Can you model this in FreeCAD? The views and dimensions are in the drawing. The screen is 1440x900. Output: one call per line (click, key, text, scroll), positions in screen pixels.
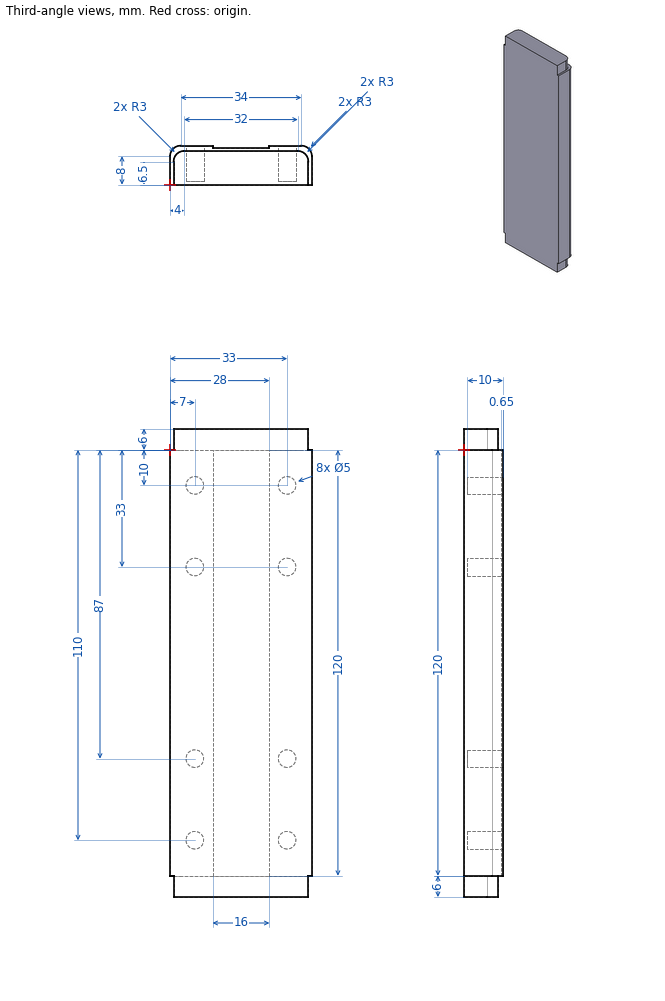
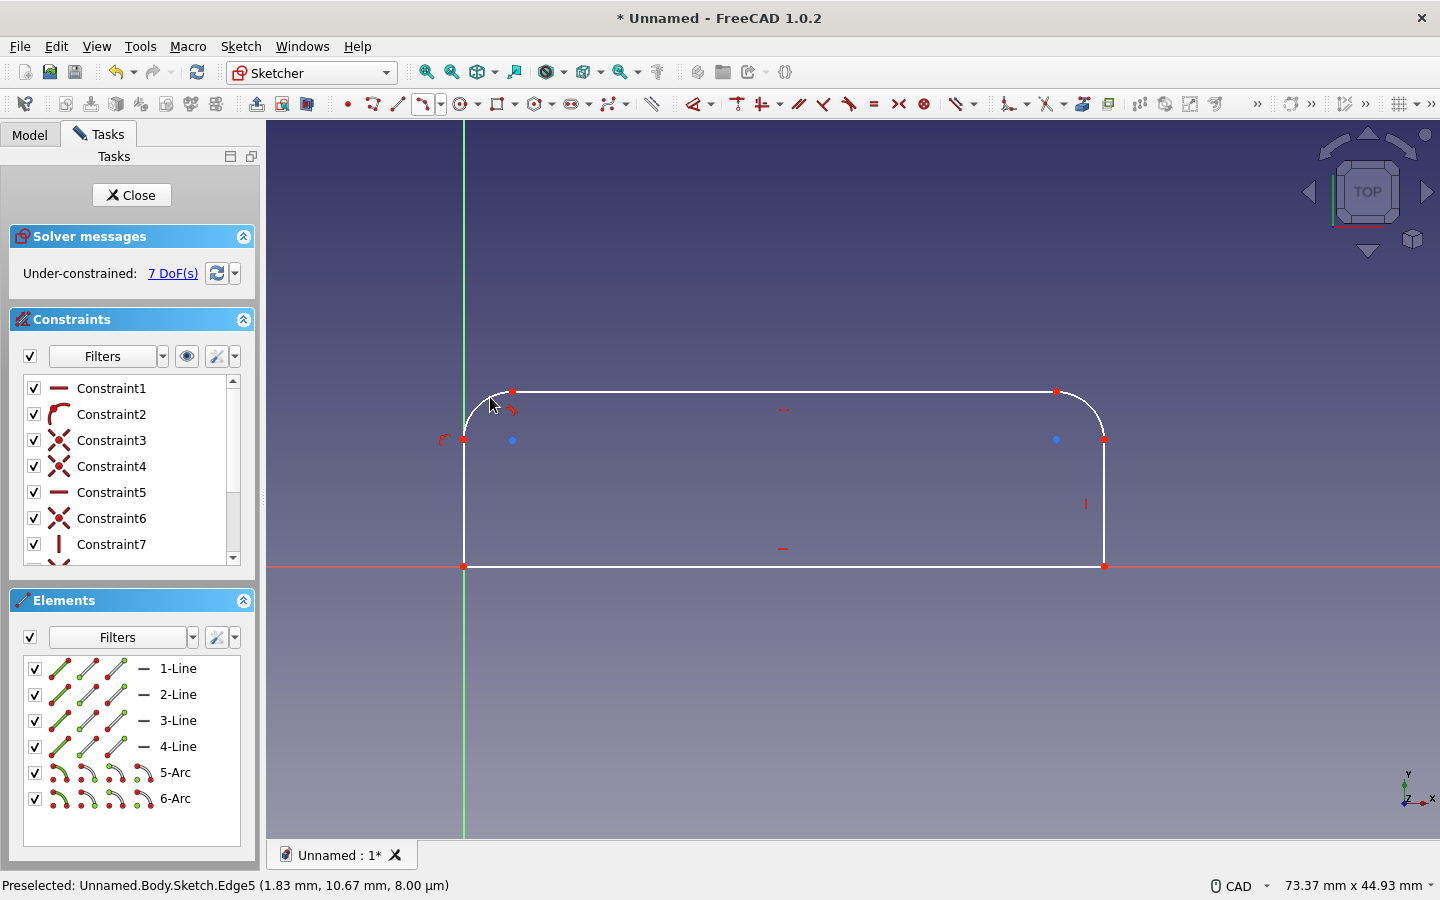
click(893, 392)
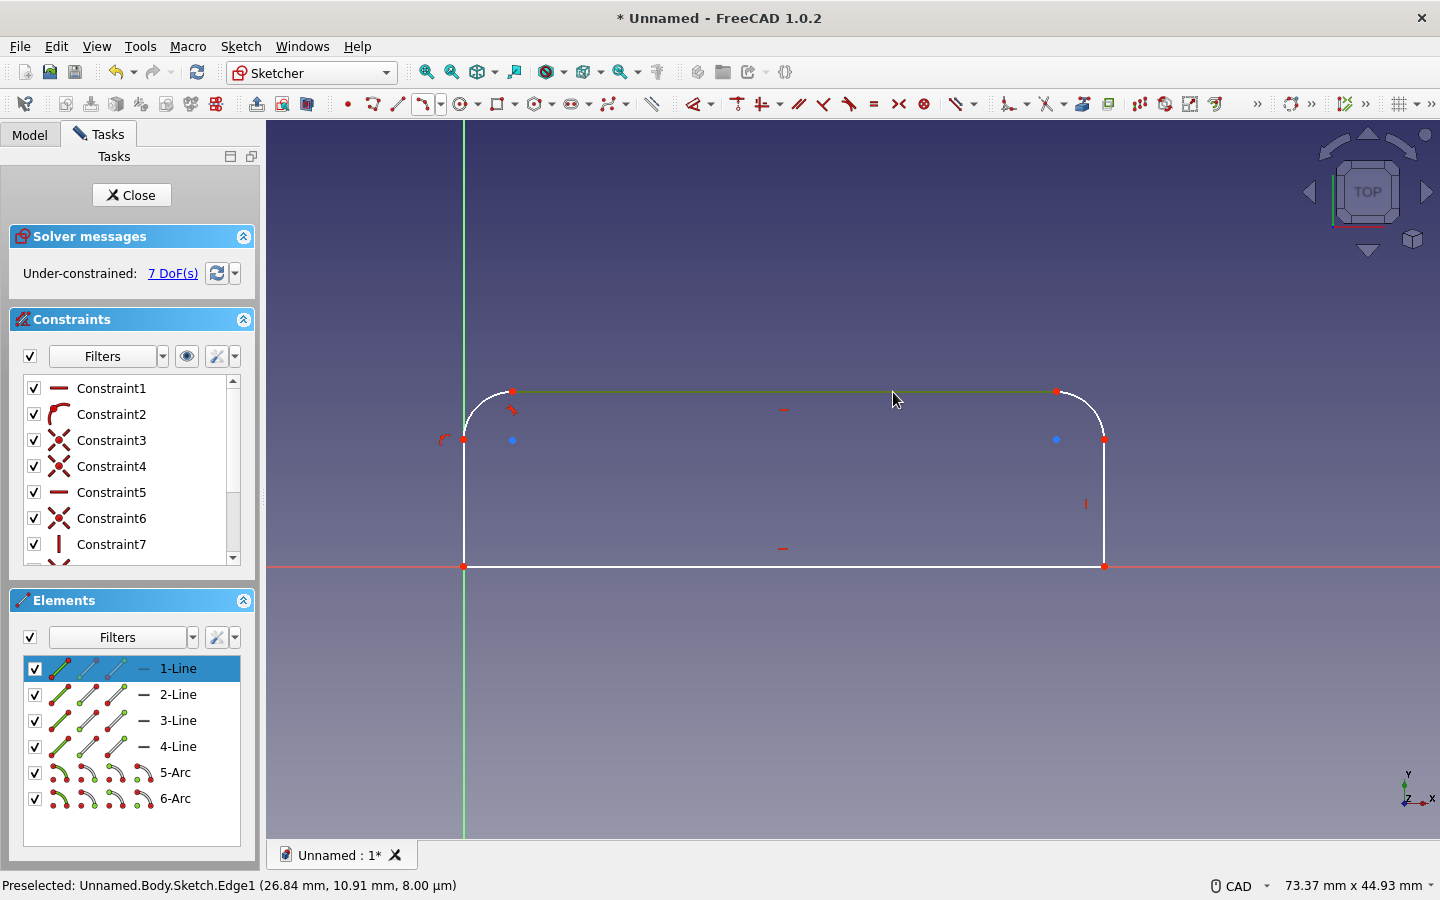
click(1099, 418)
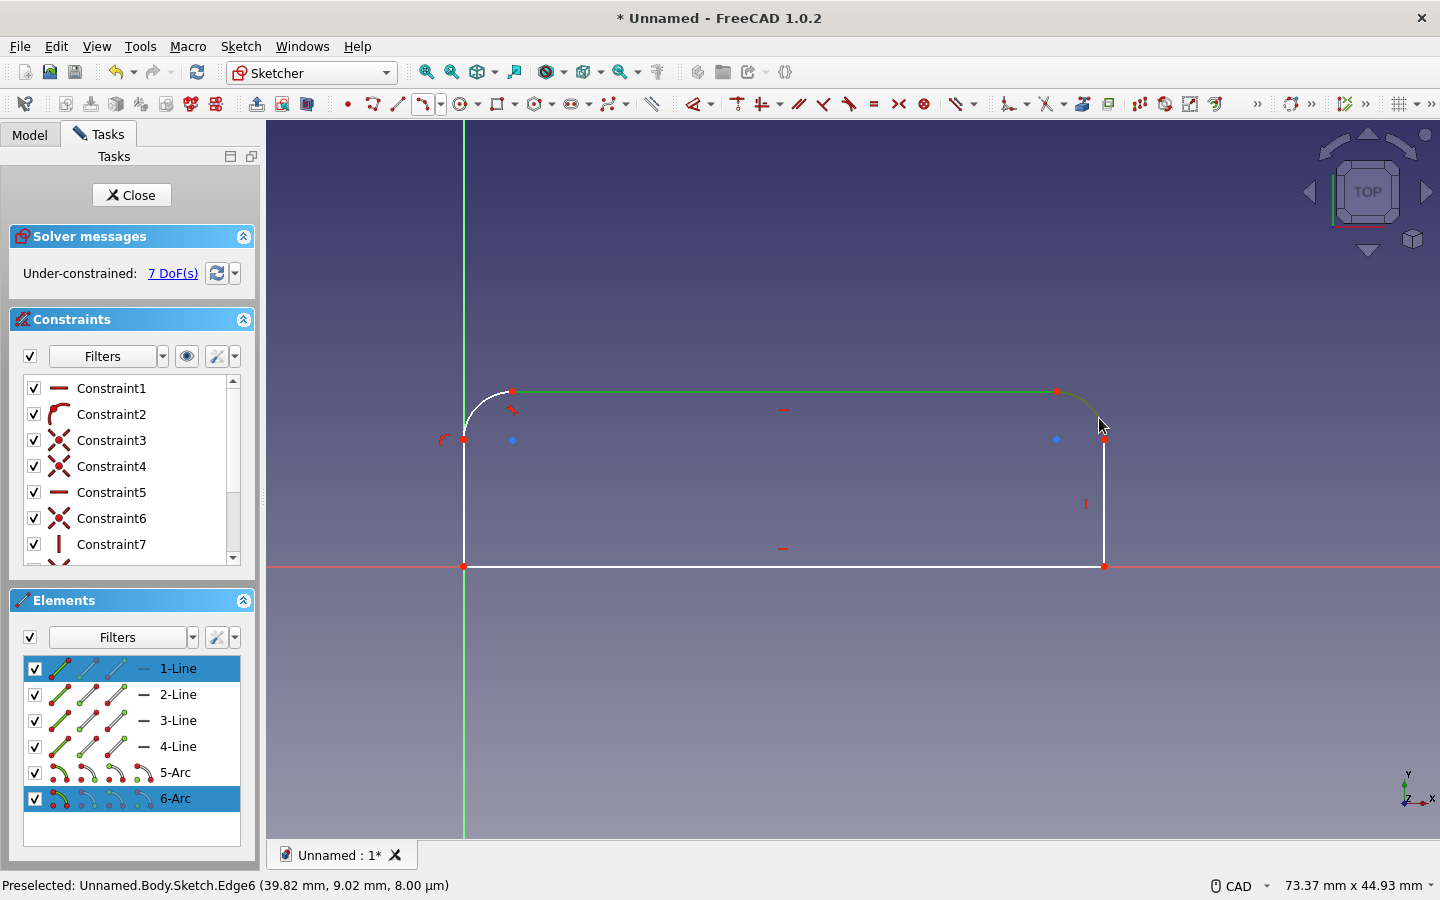
key(t)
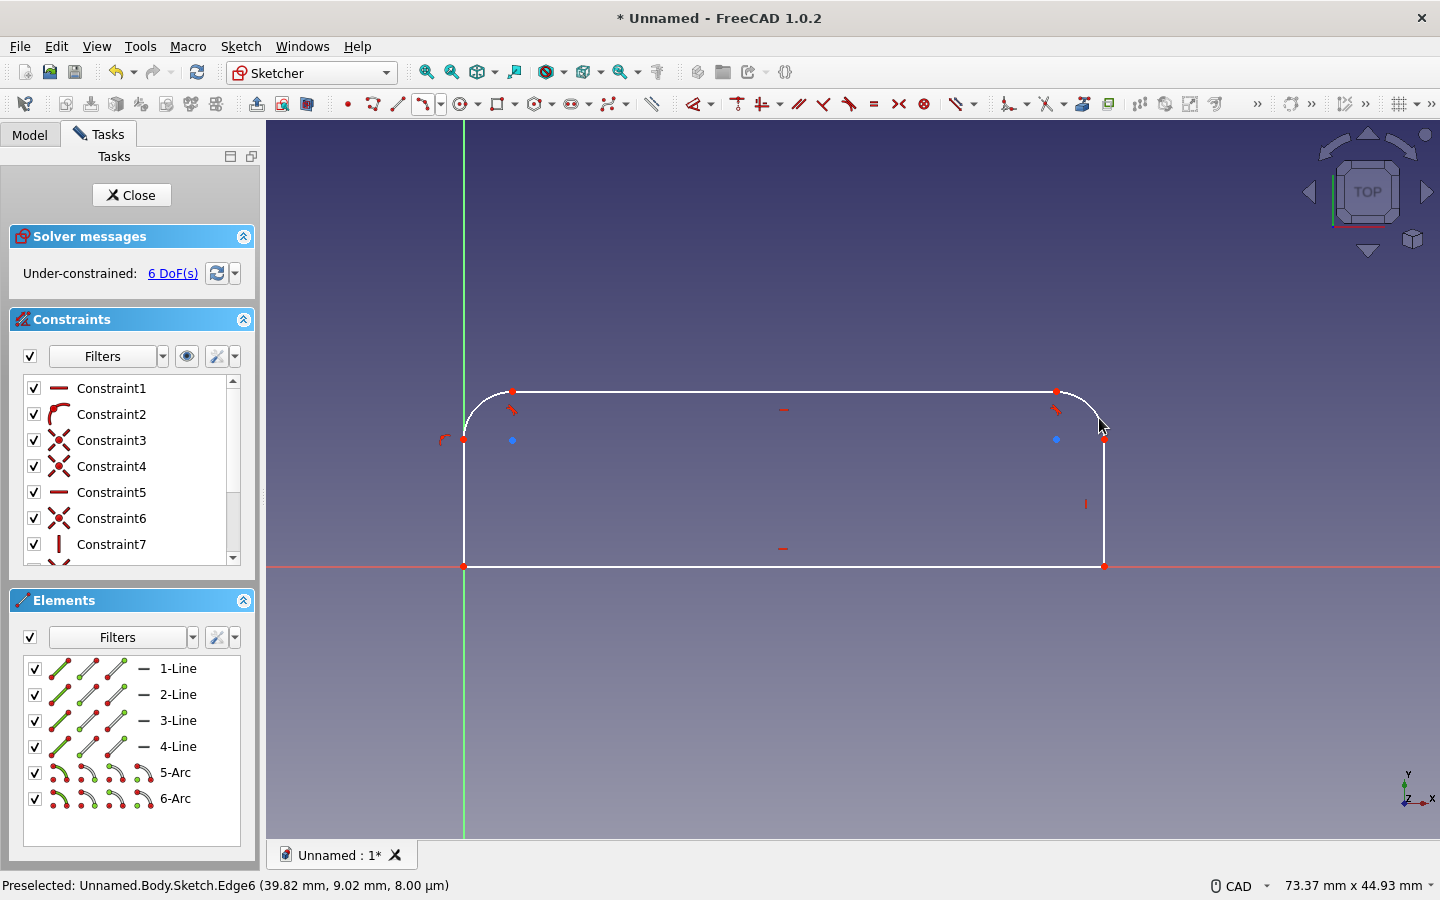
click(464, 478)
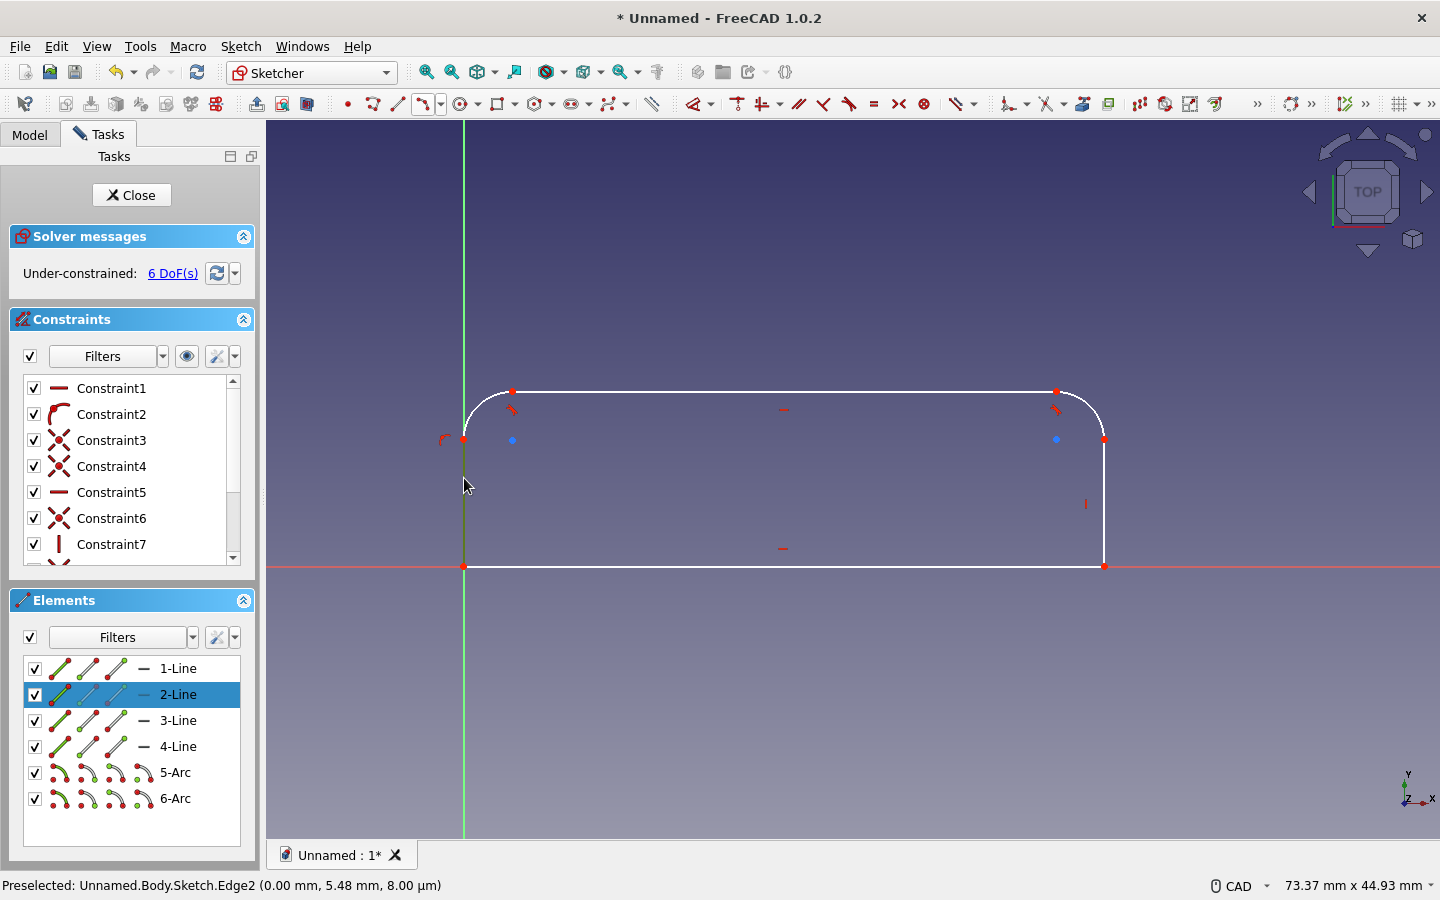
click(490, 397)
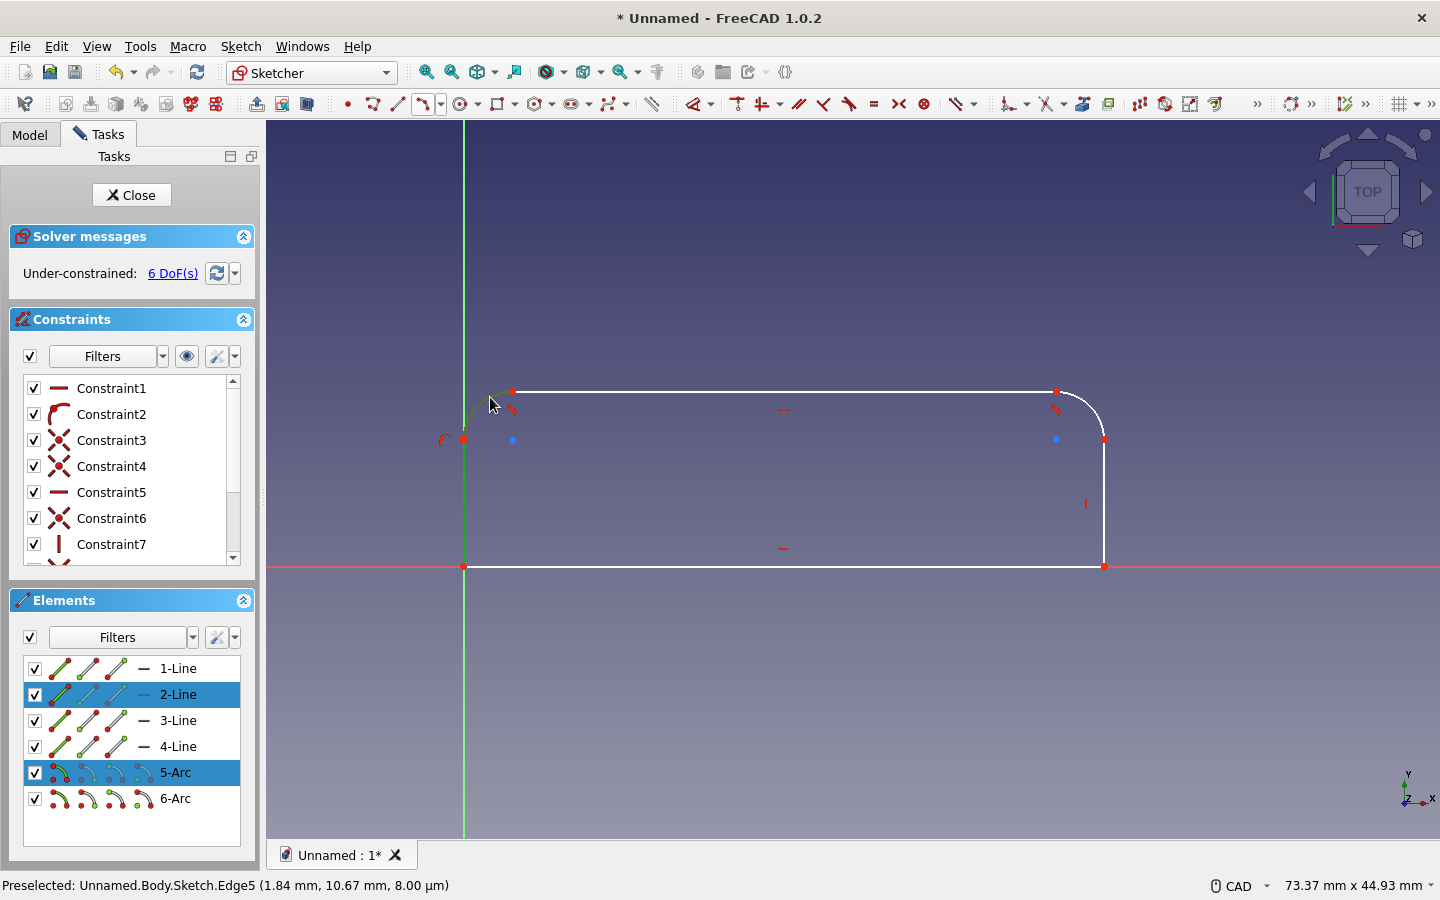
click(849, 104)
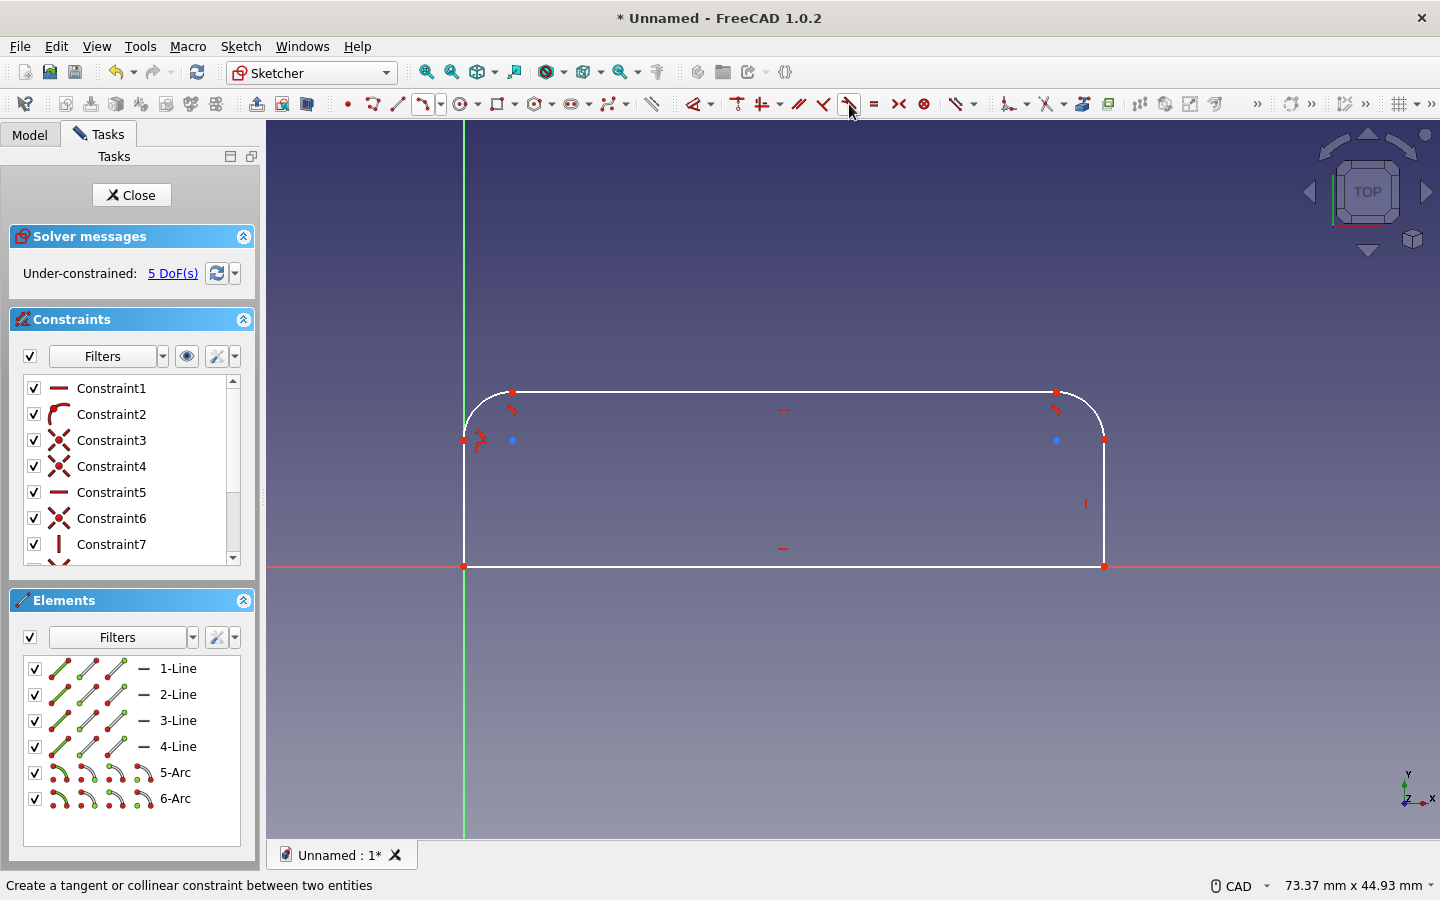
click(1104, 529)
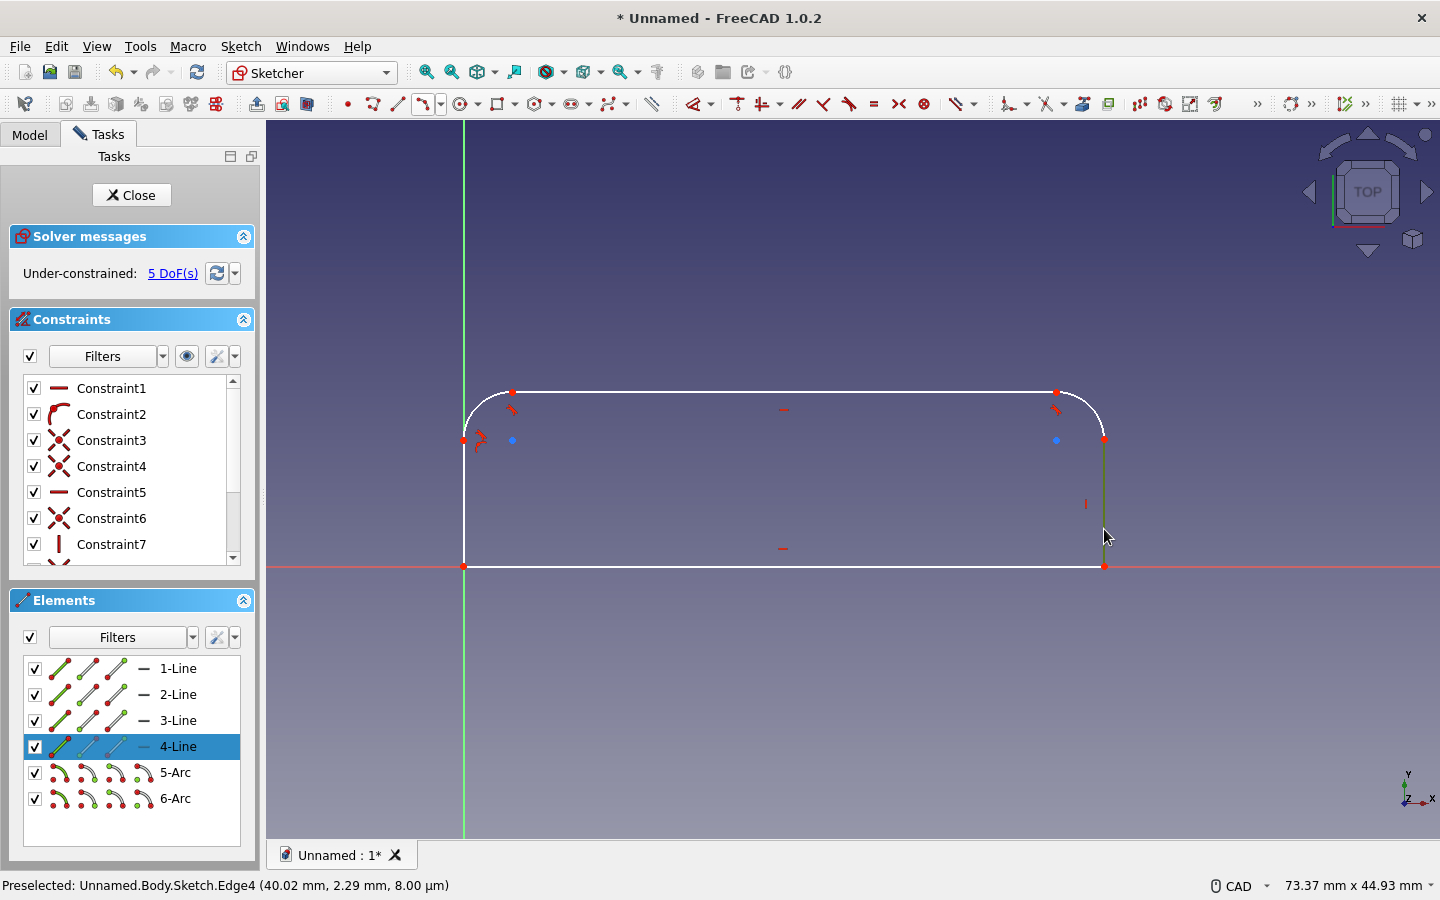
click(1099, 418)